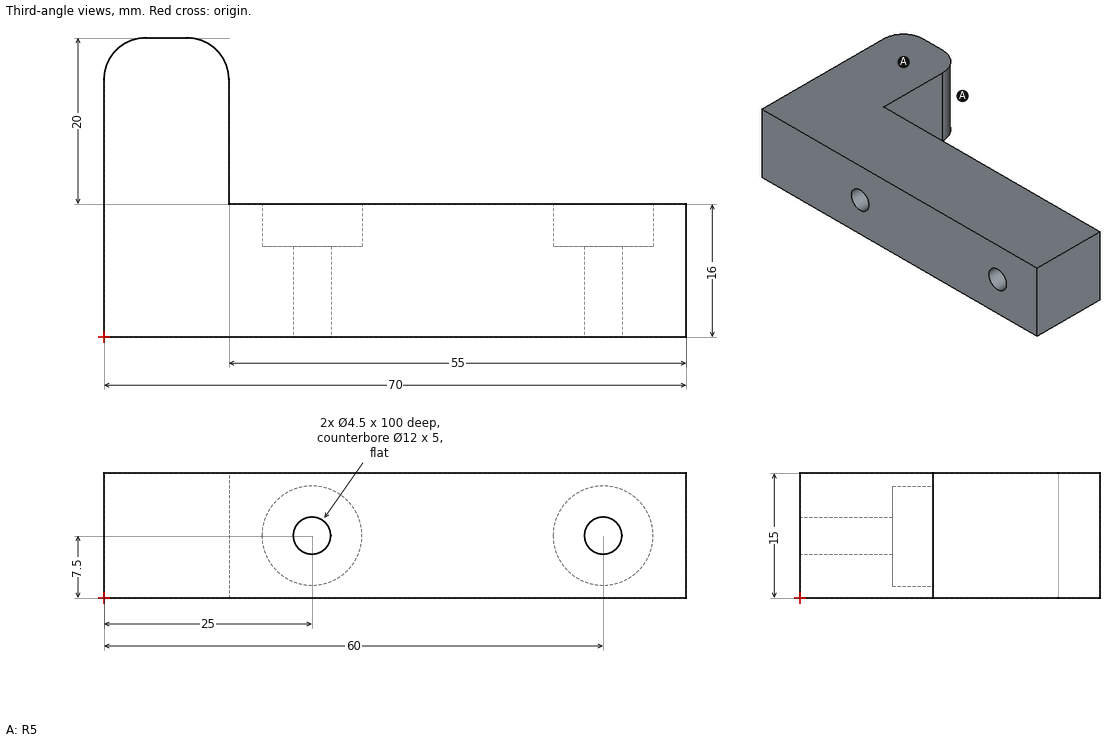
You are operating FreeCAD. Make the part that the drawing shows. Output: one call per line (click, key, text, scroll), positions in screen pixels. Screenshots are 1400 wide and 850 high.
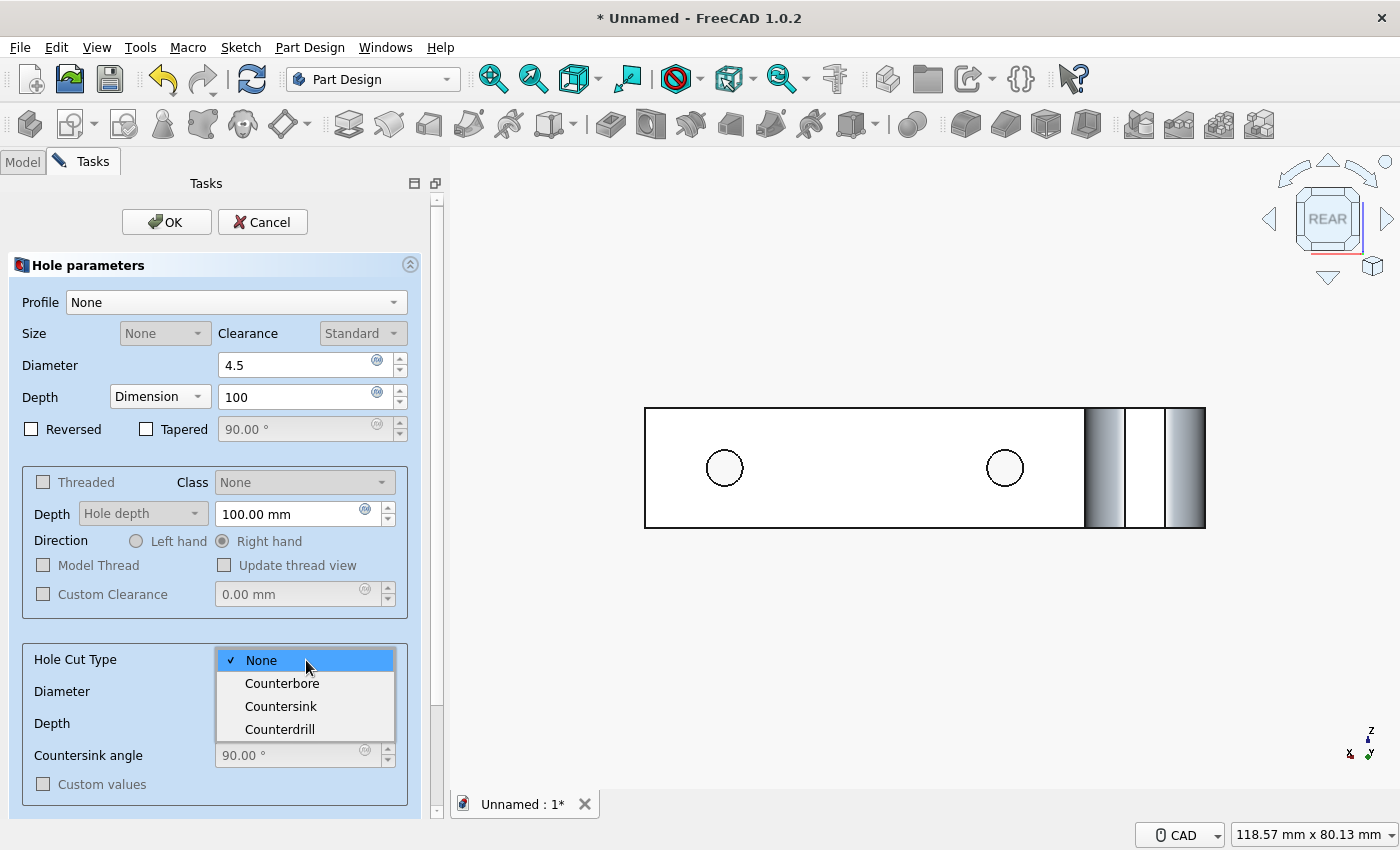
click(304, 684)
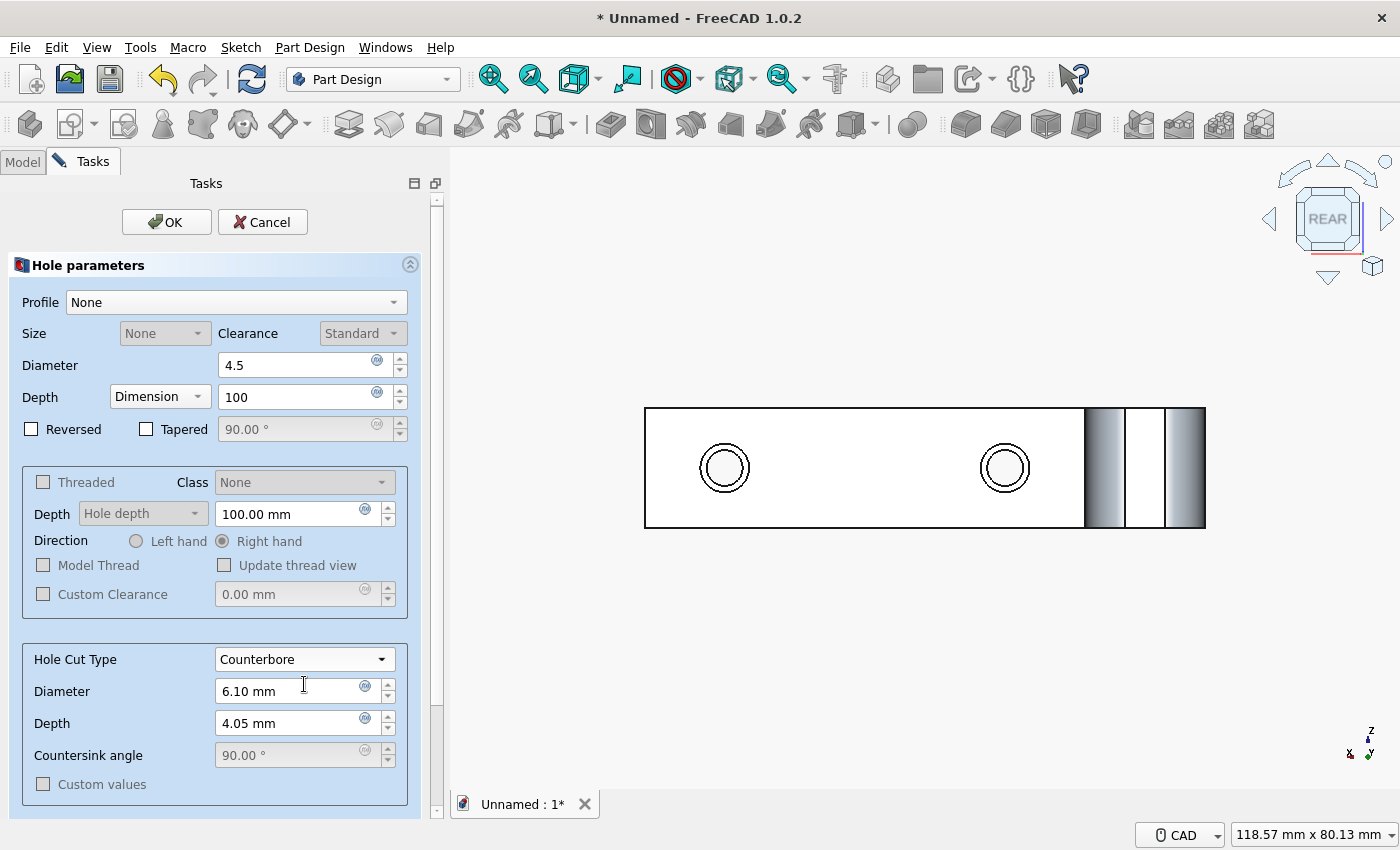
triple_click(298, 691)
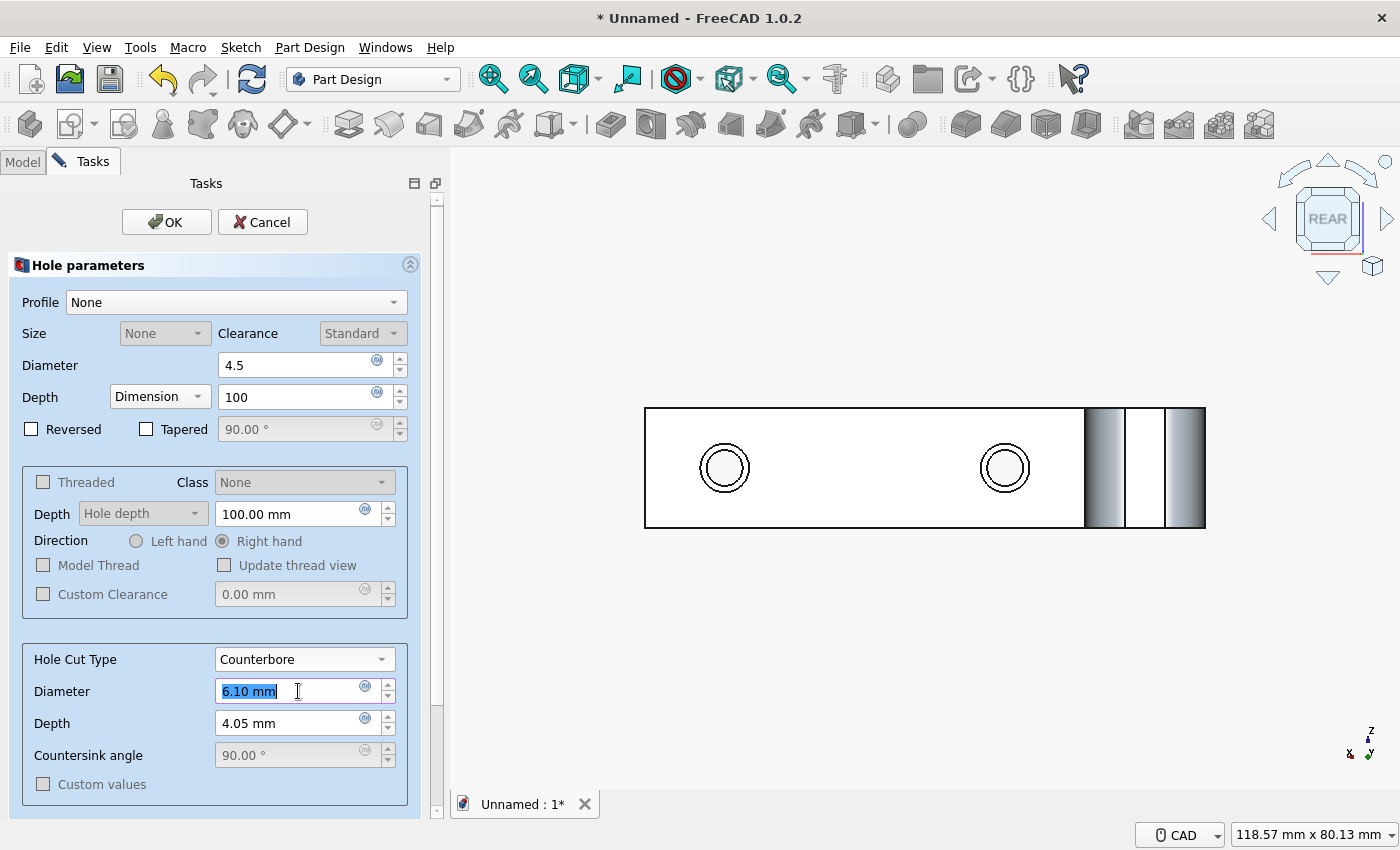
text(12)
key(Tab)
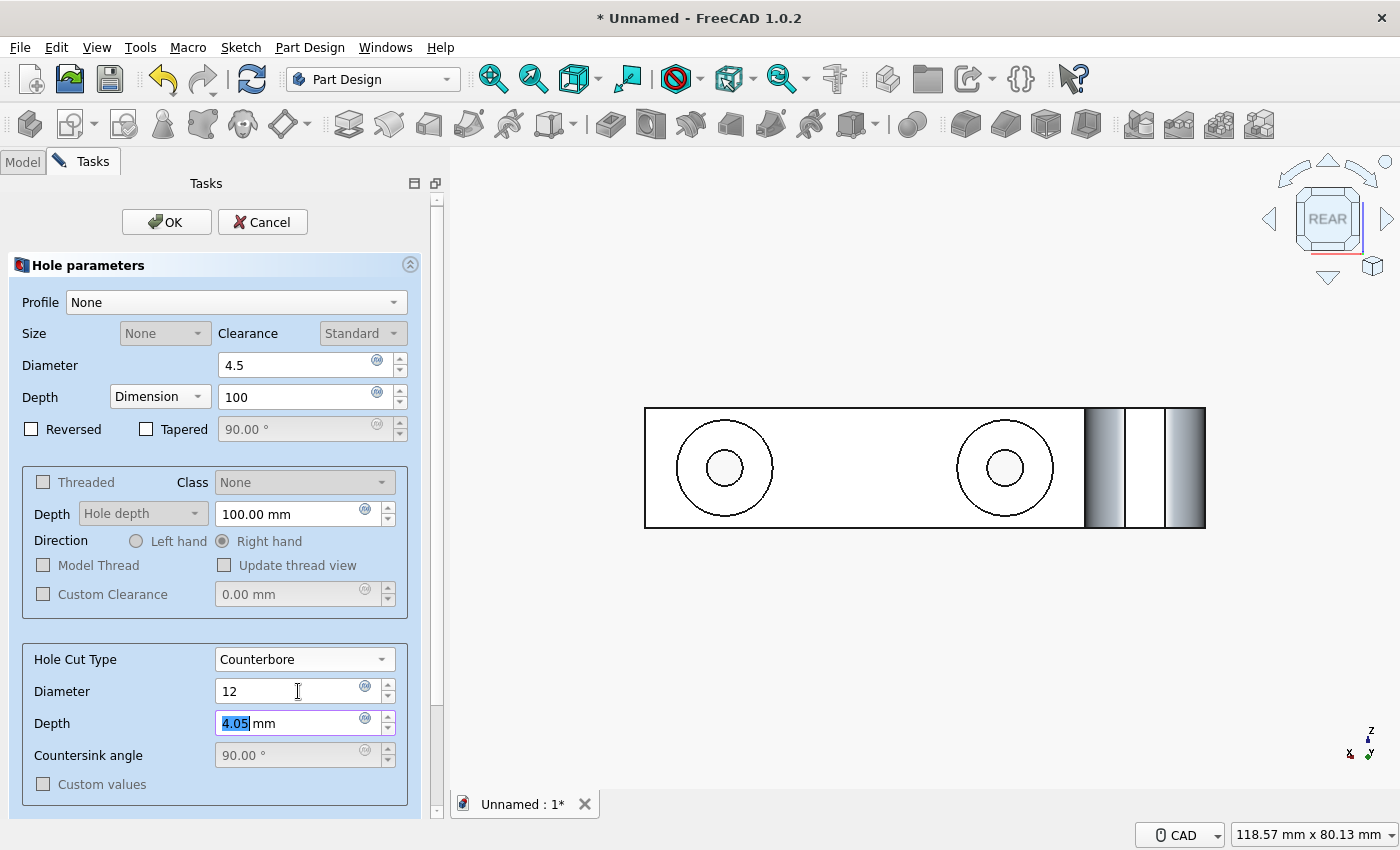
text(5)
key(Tab)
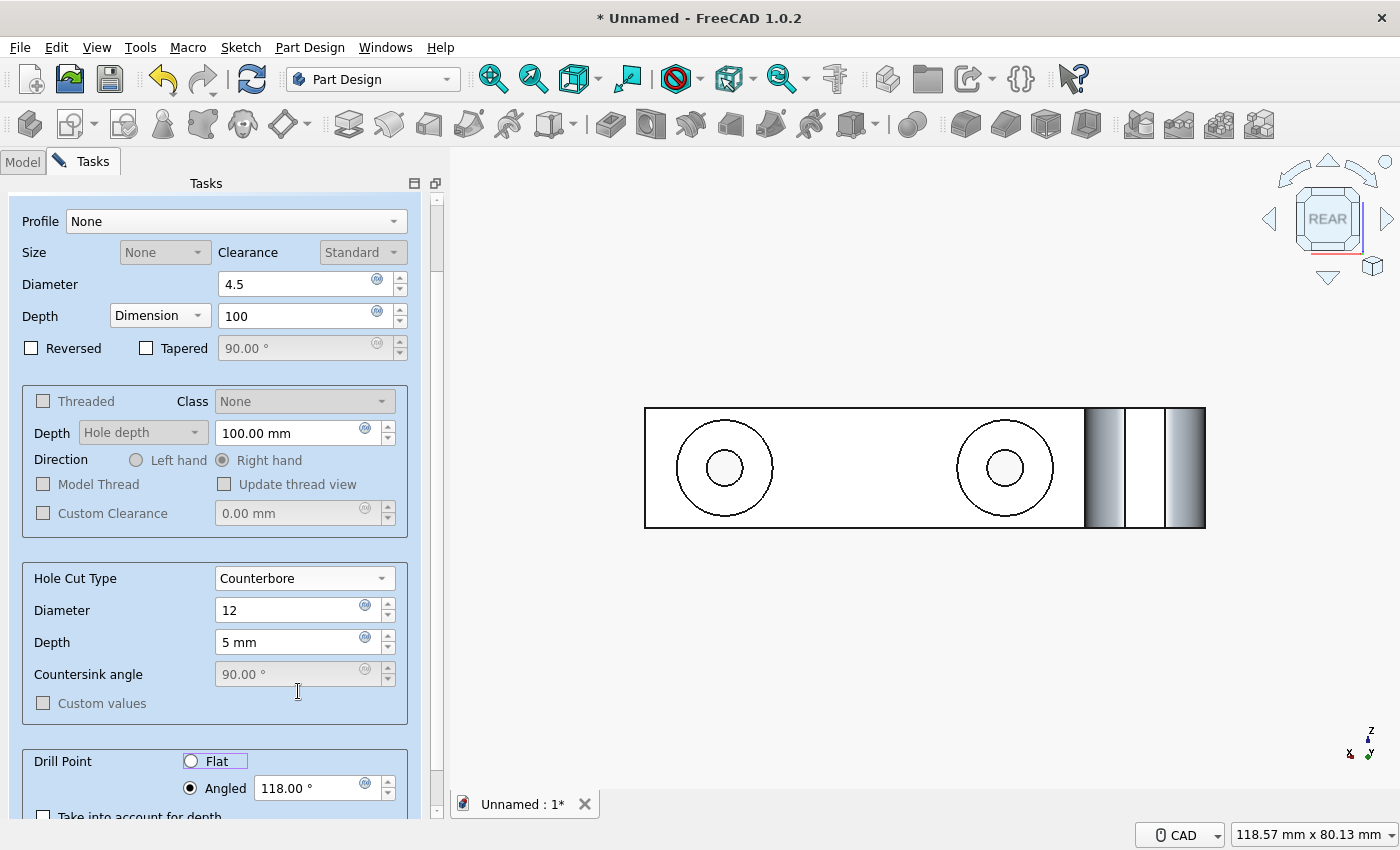
click(191, 761)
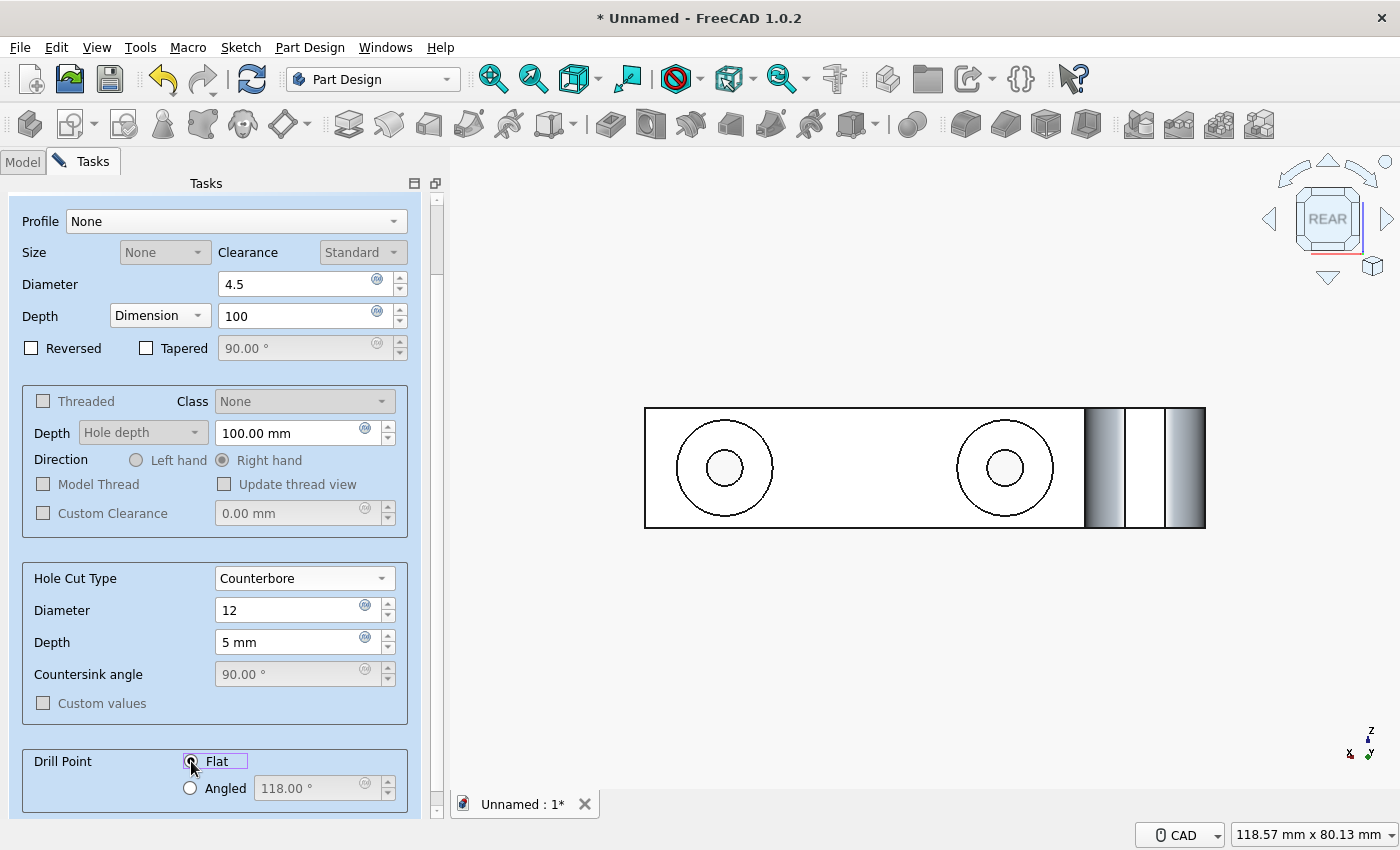
scroll(437, 506, up, 3)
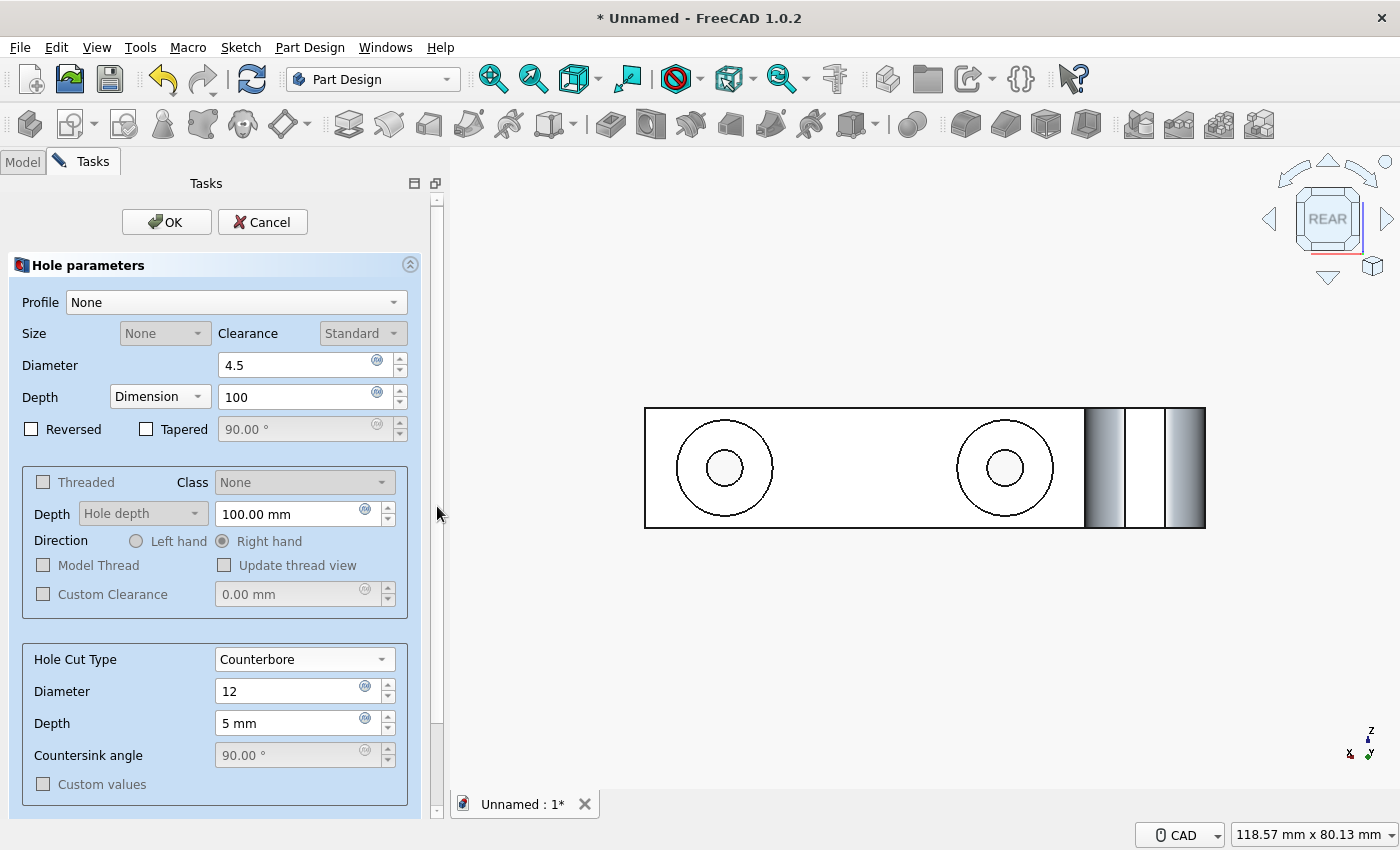
click(167, 222)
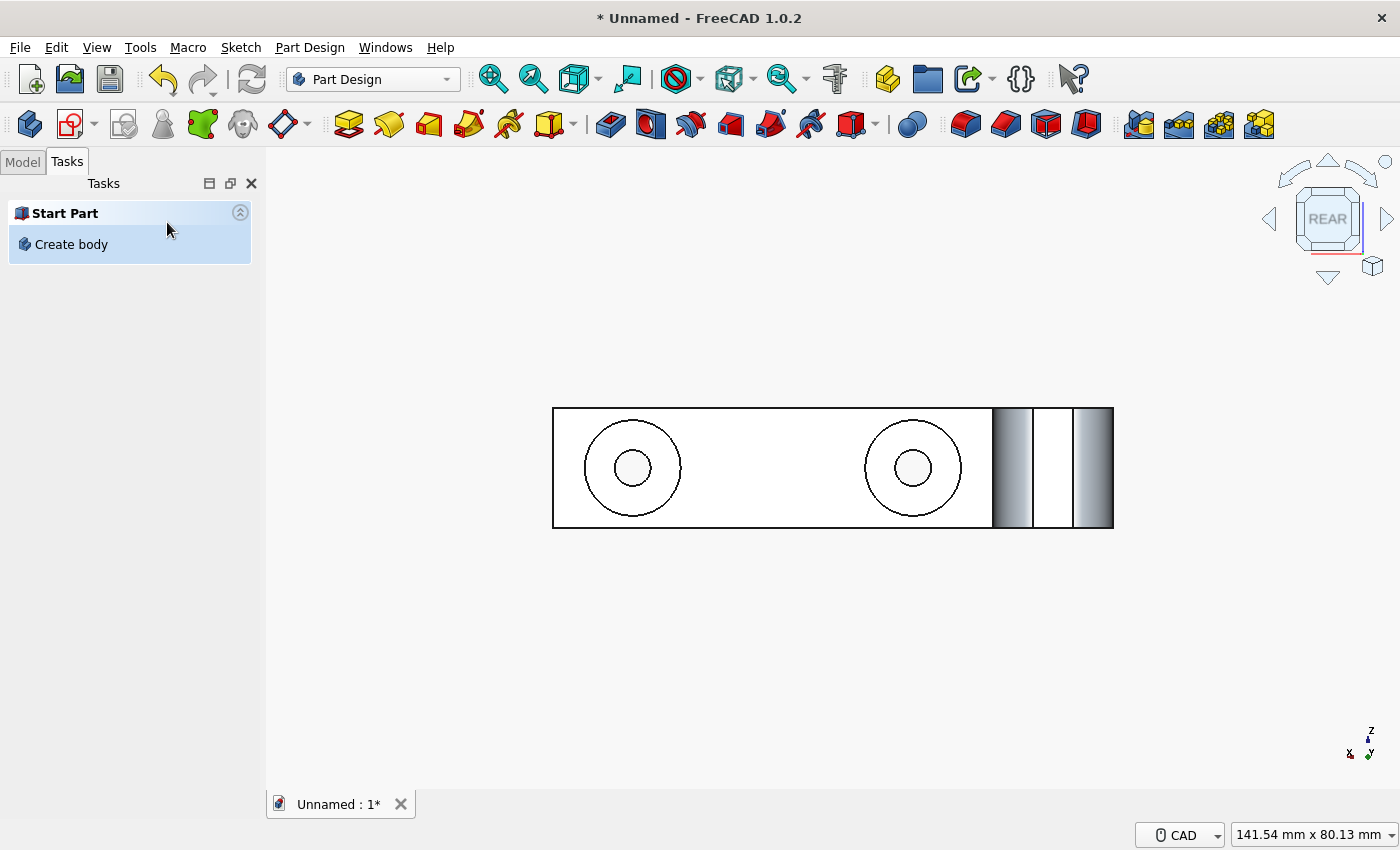
key(0)